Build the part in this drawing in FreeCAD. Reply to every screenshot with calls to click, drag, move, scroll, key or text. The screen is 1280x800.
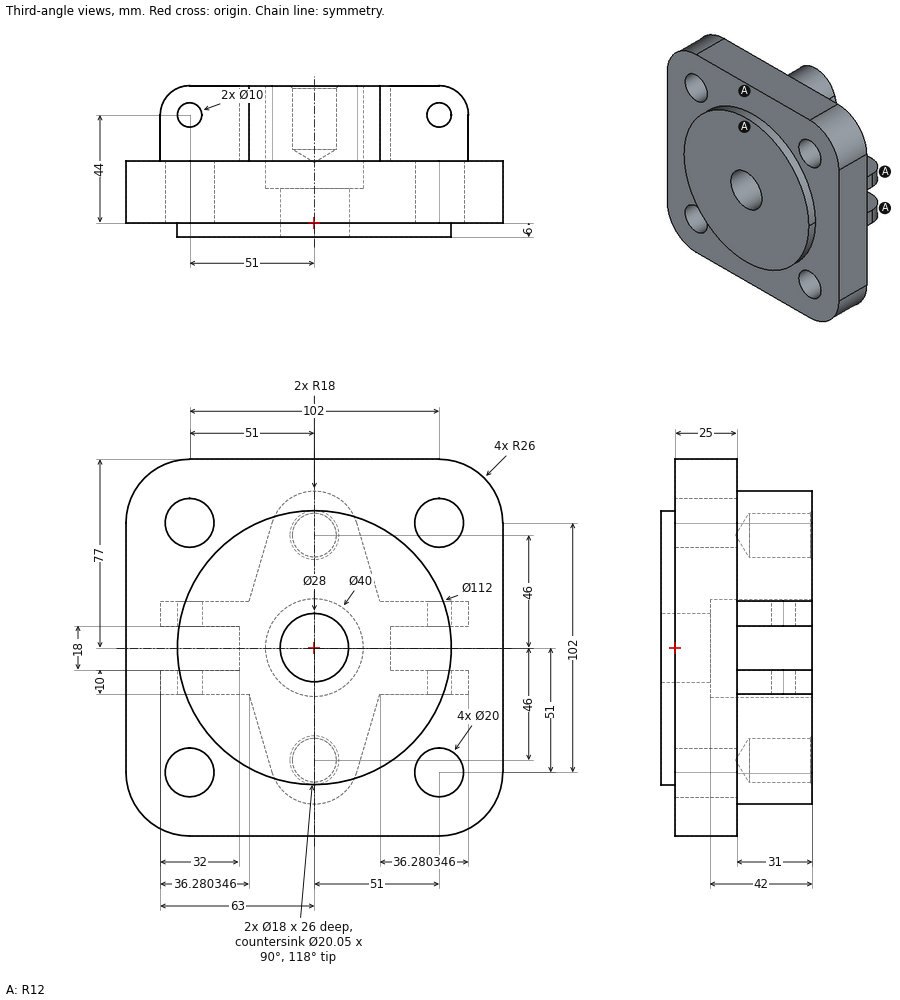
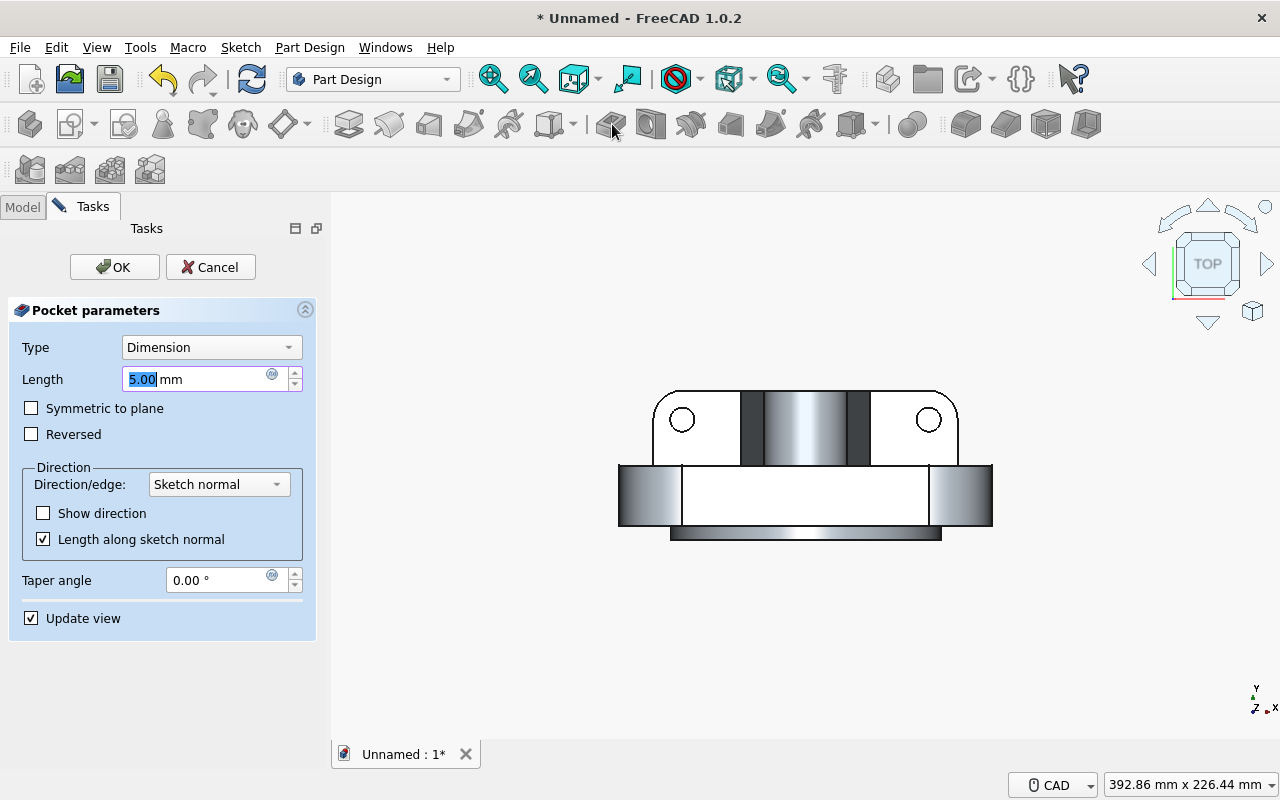
click(212, 348)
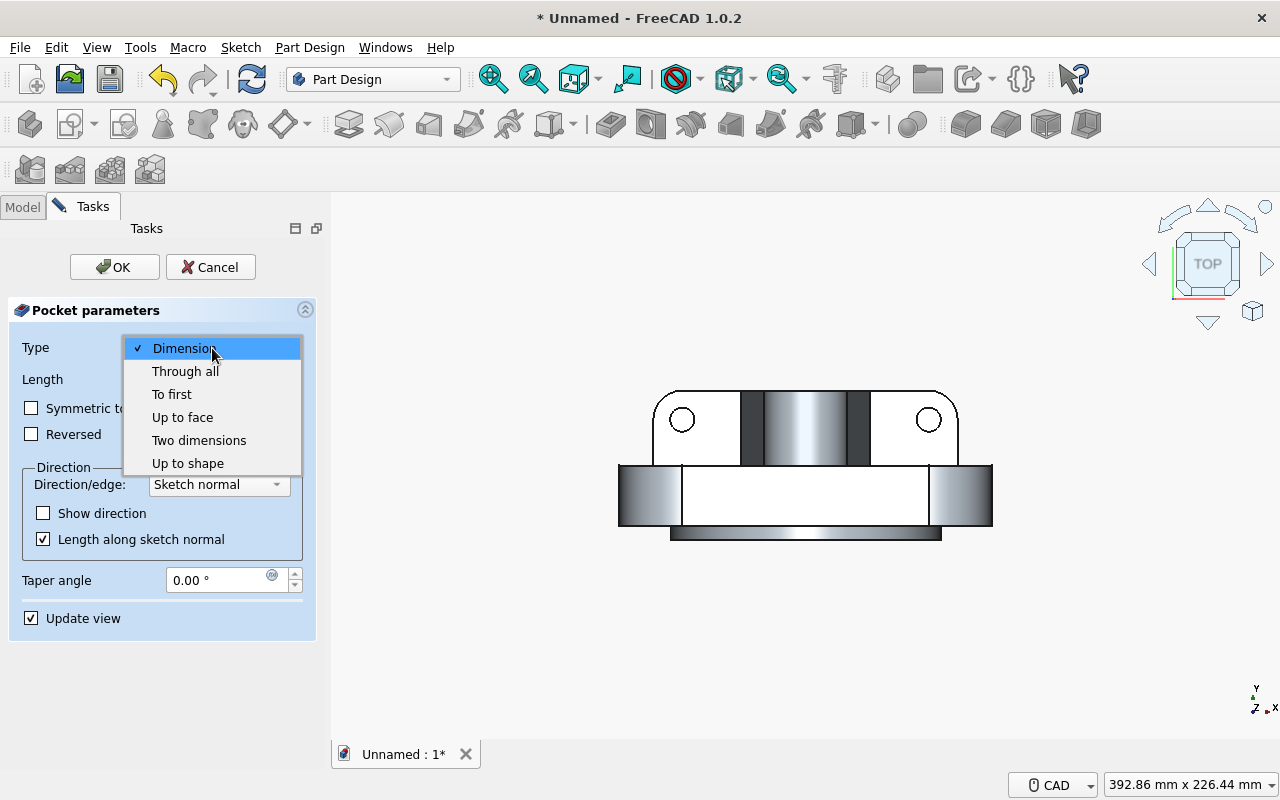
click(212, 372)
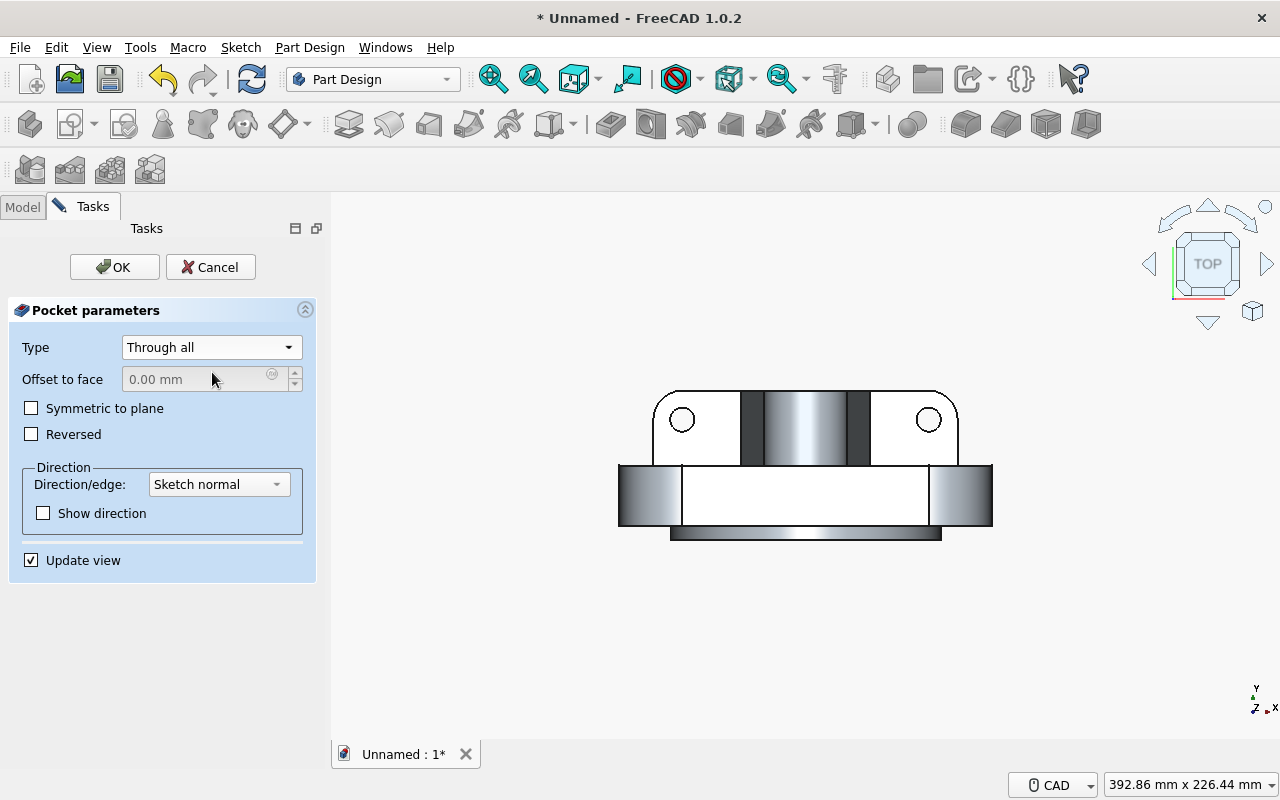
click(115, 267)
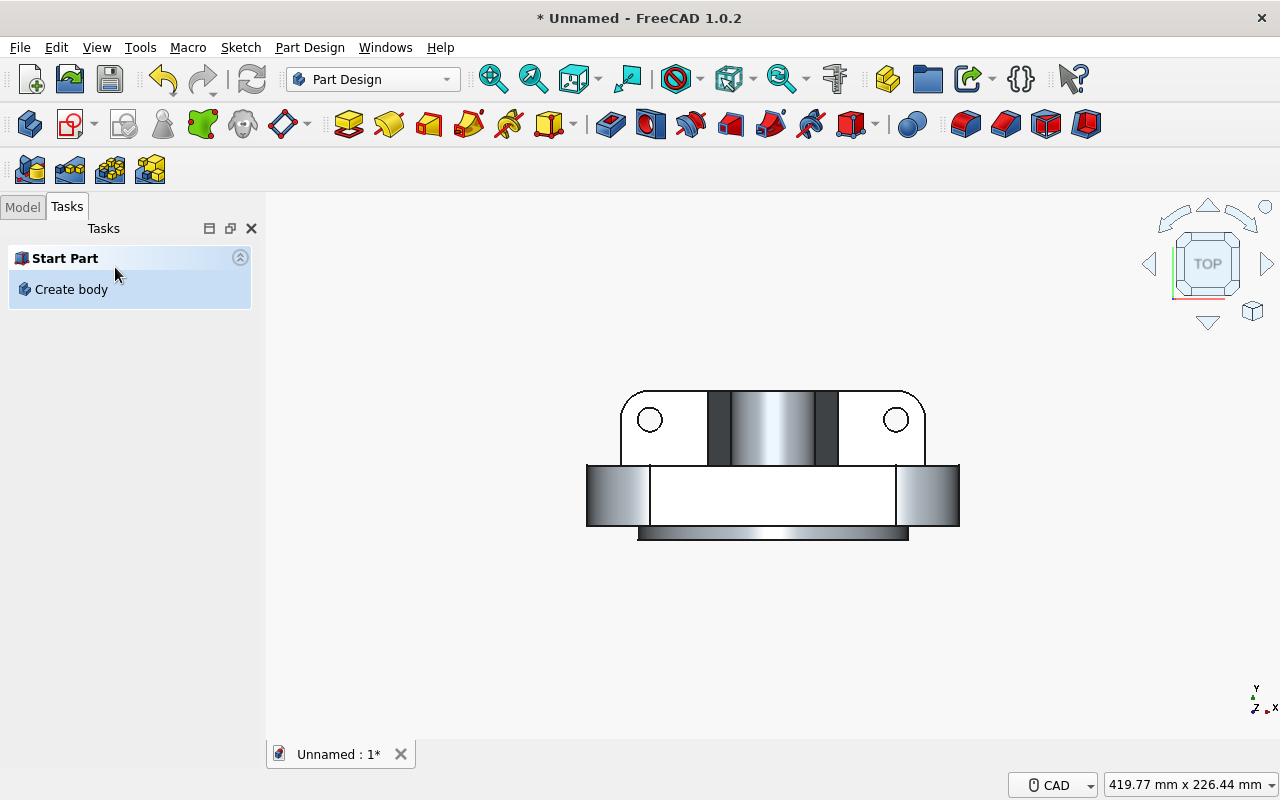
key(v)
key(f)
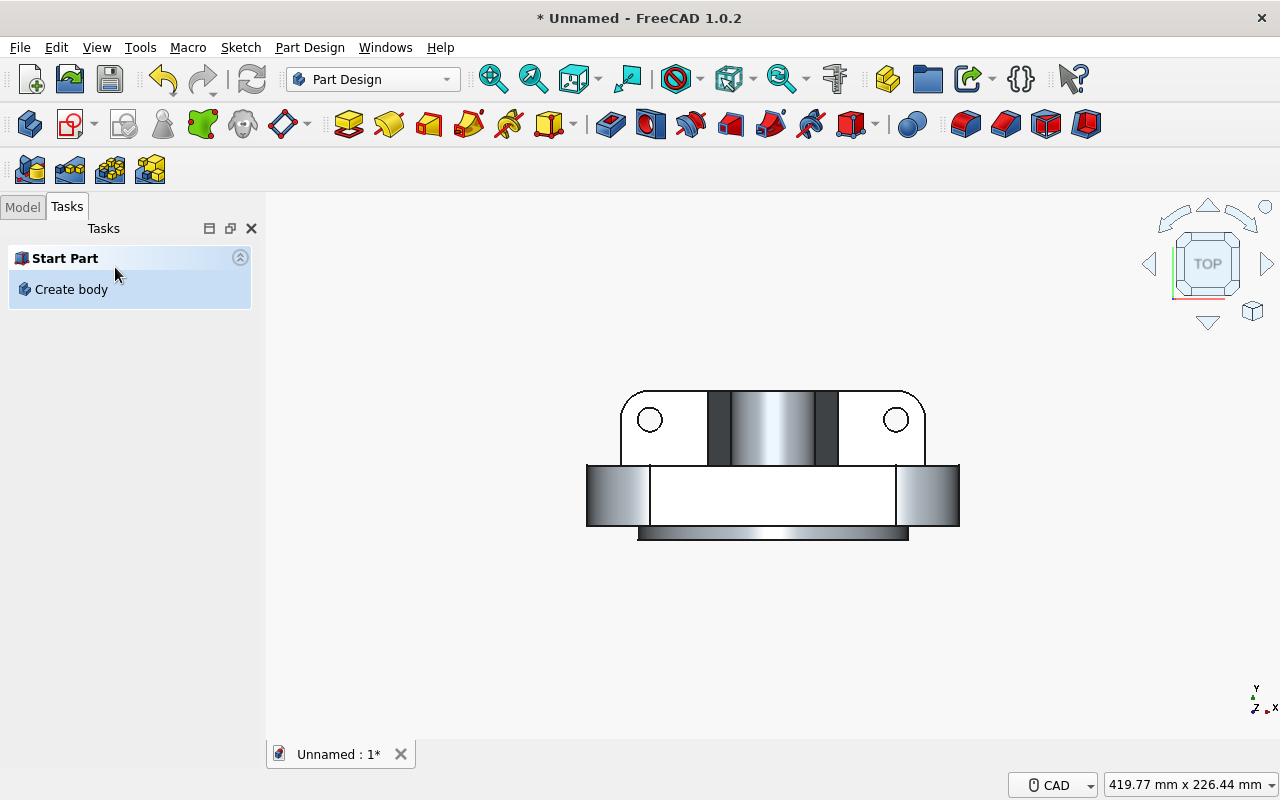
key(4)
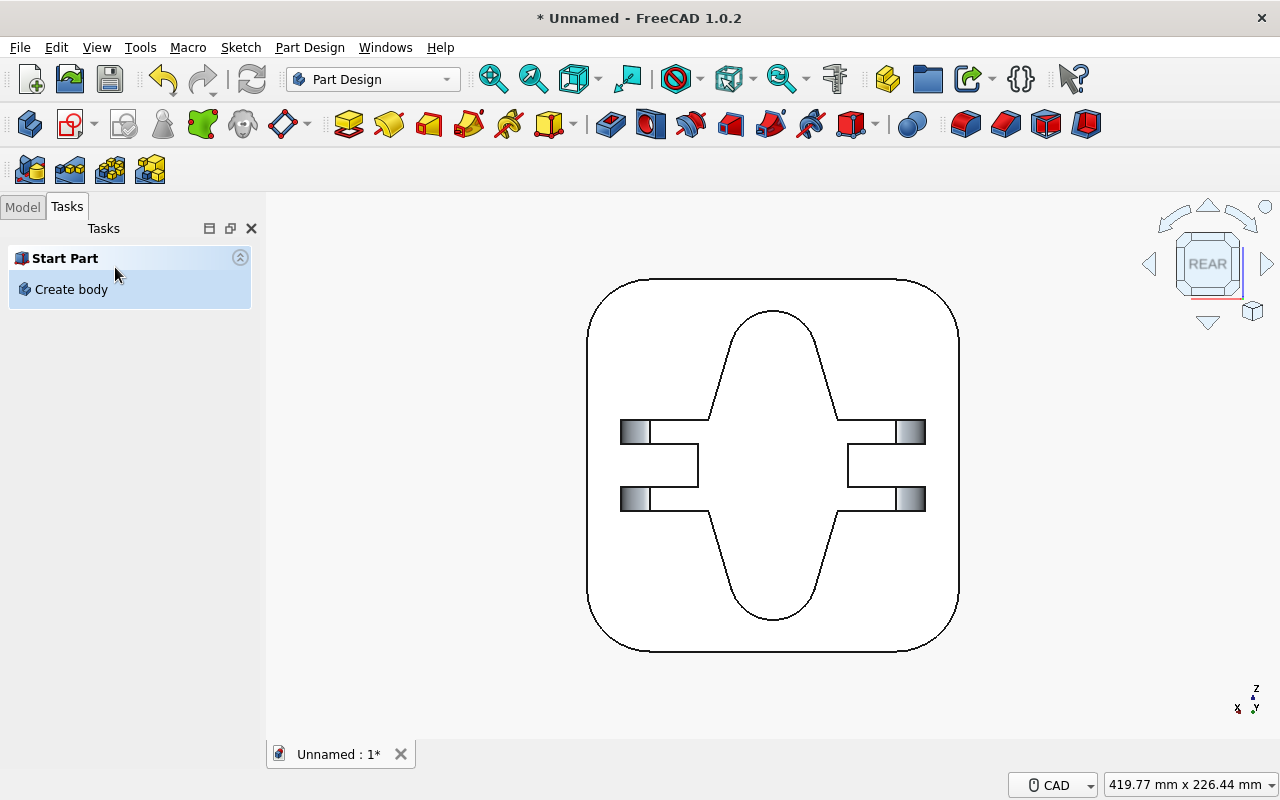
click(773, 464)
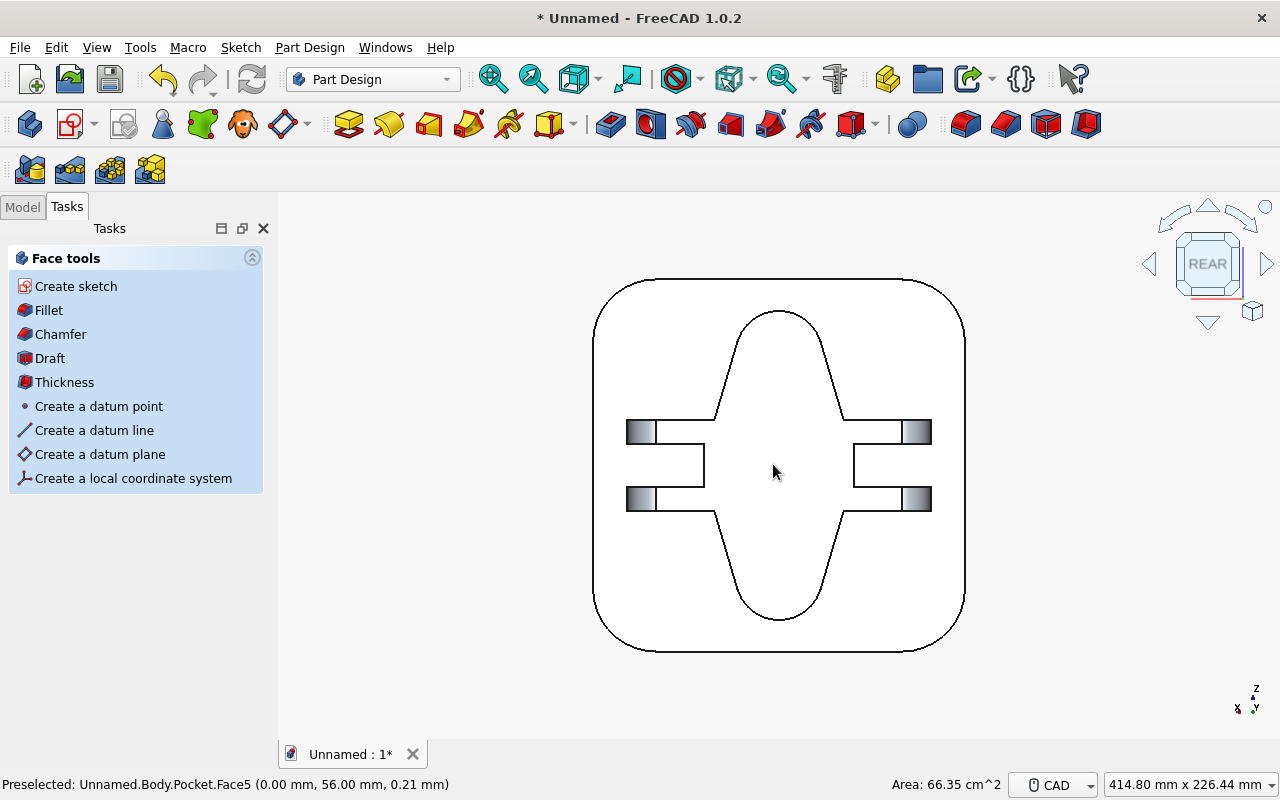
click(70, 124)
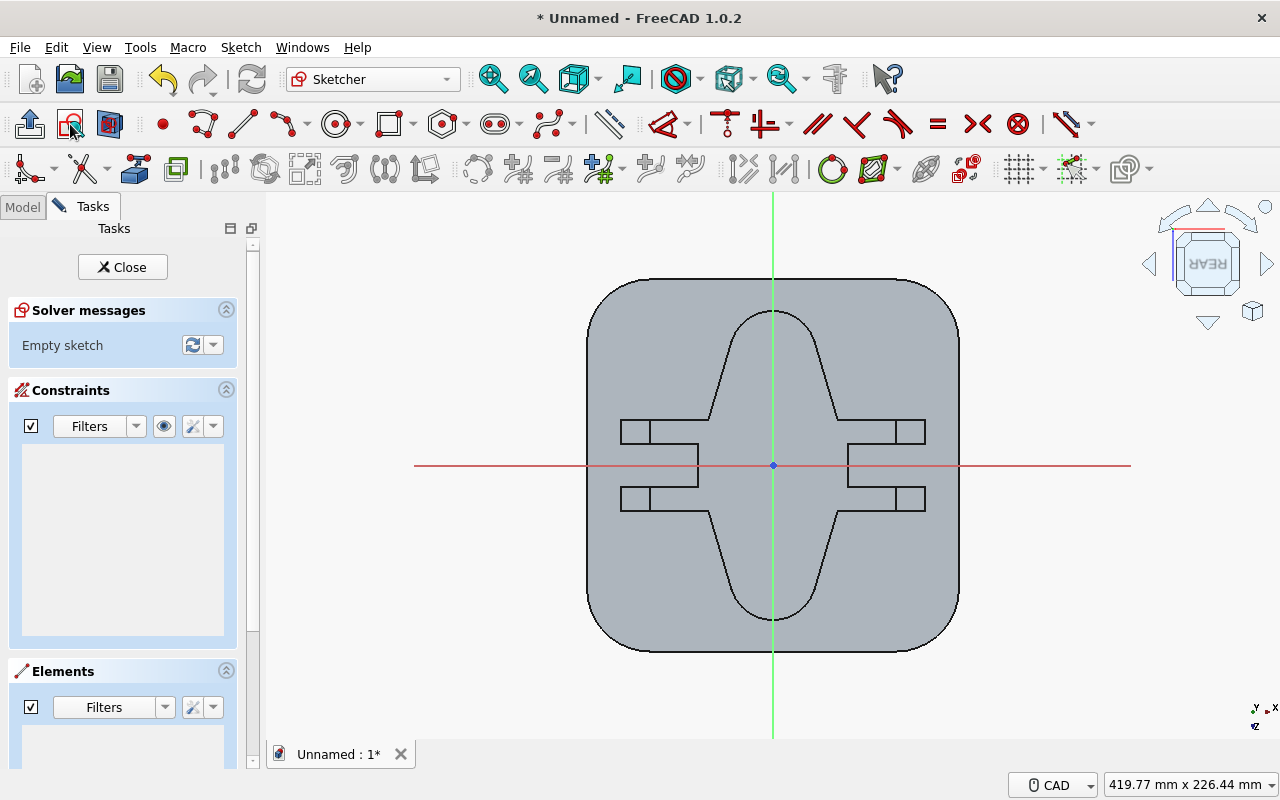
scroll(803, 466, up, 6)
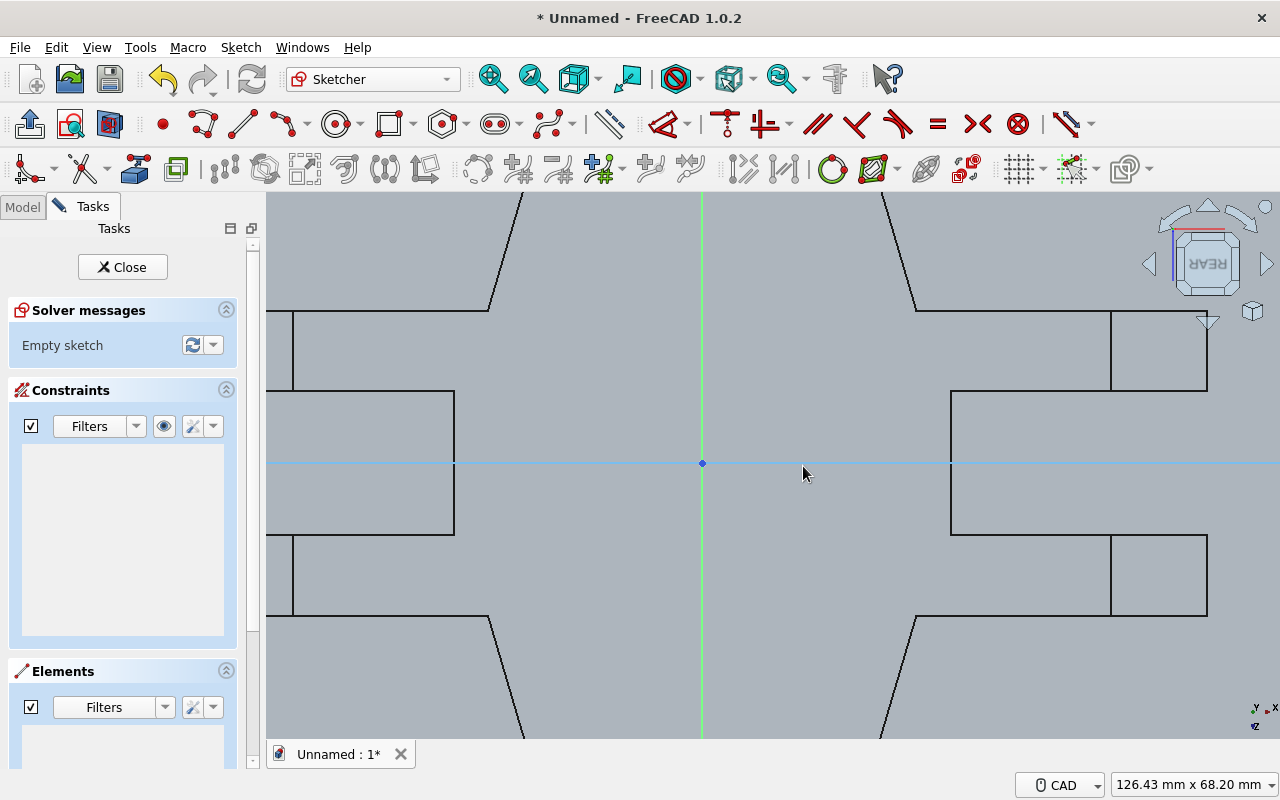
click(336, 124)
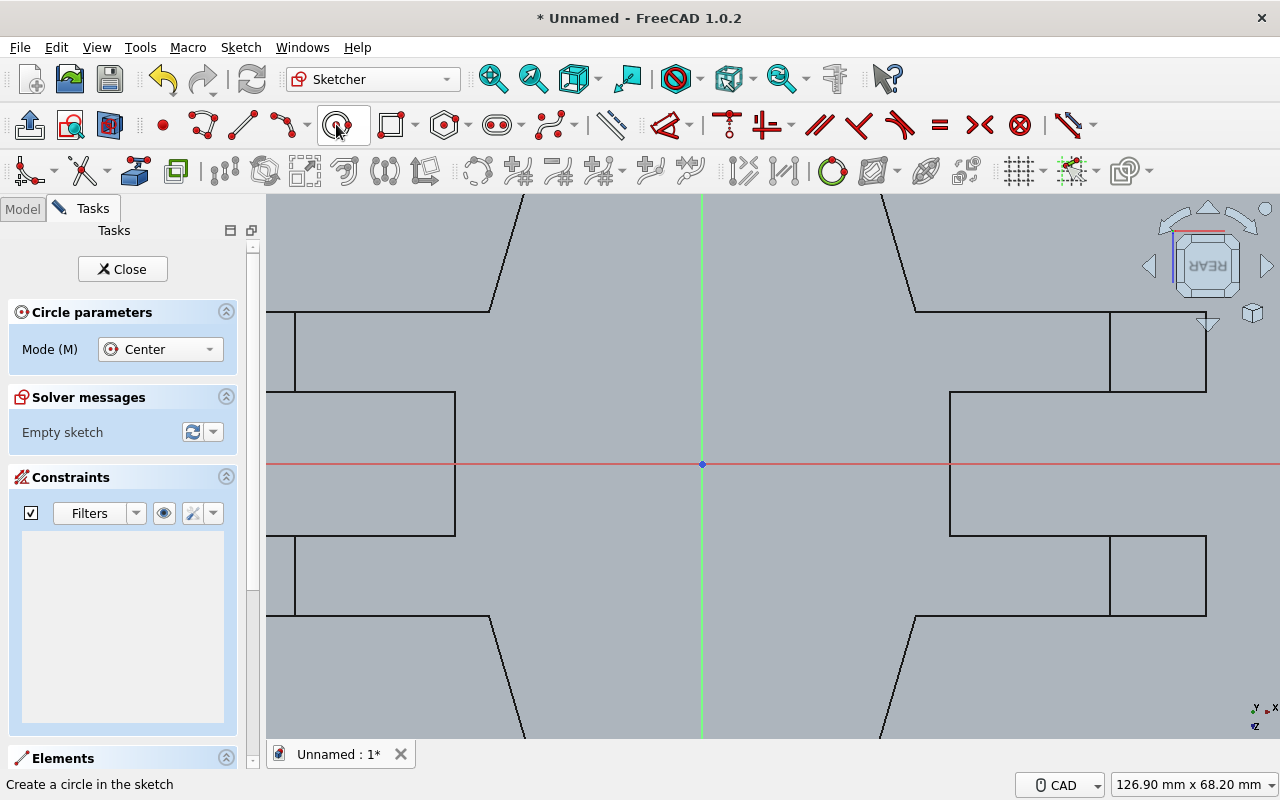
click(702, 464)
click(815, 351)
key(Escape)